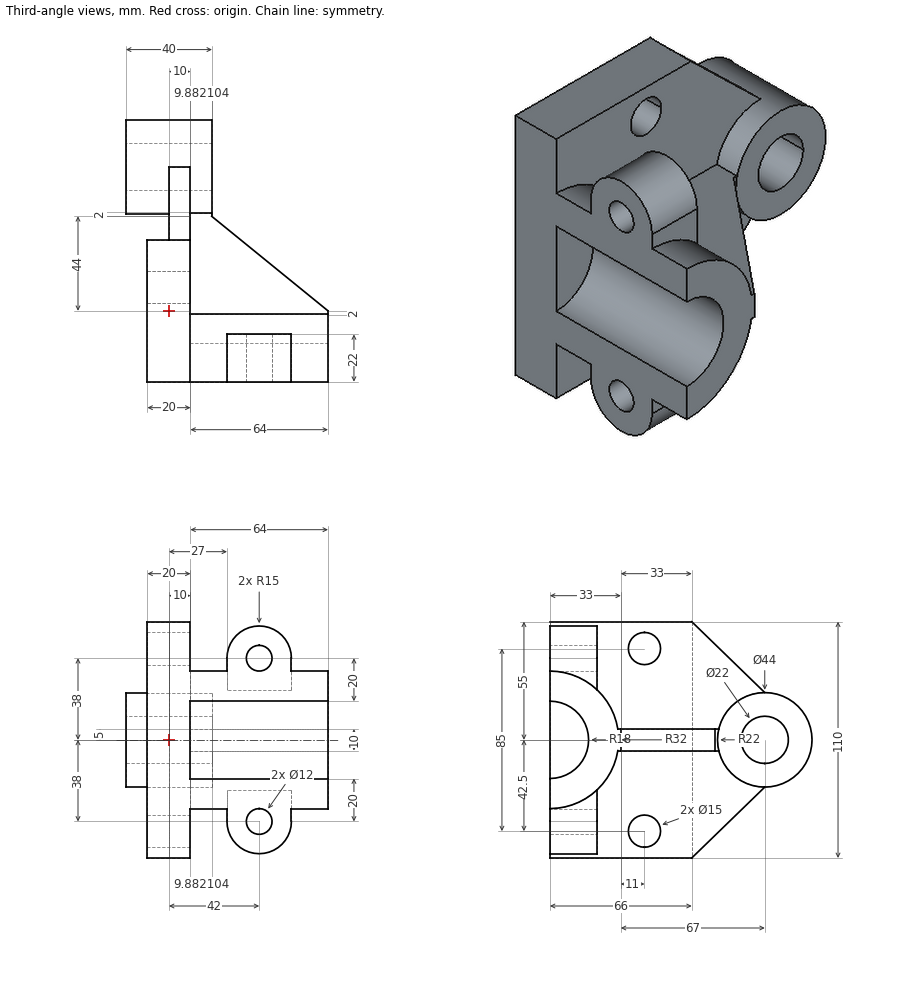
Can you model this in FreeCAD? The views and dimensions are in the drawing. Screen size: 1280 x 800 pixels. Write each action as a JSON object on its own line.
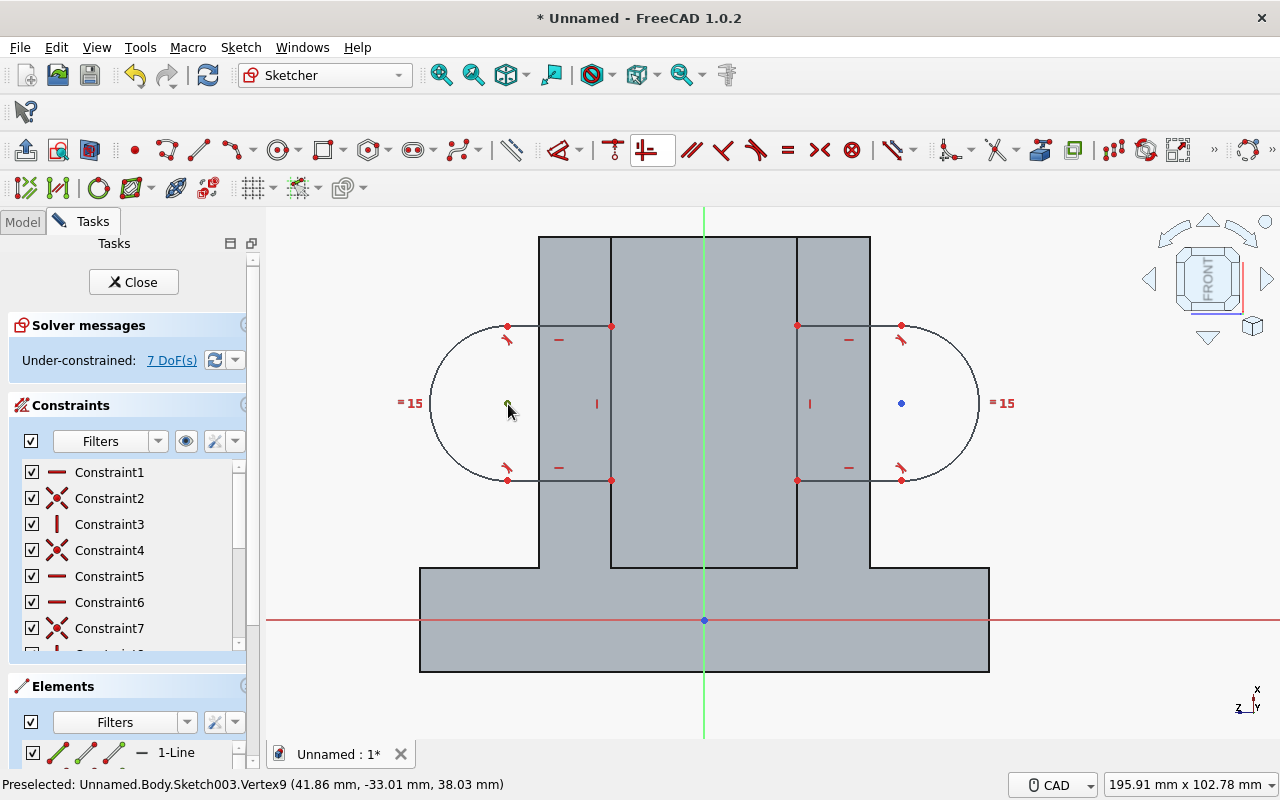
{"action": "left_click", "coordinate": [901, 403]}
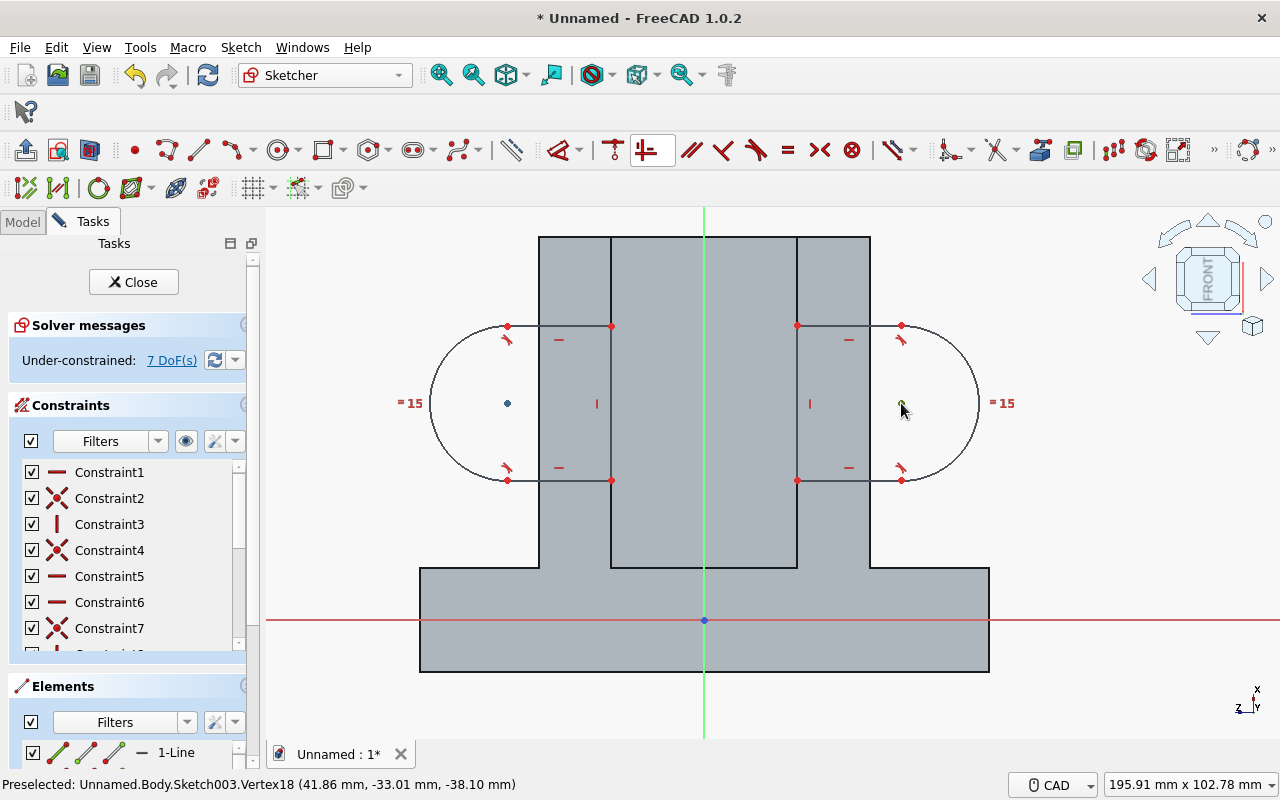
{"action": "left_click", "coordinate": [704, 677]}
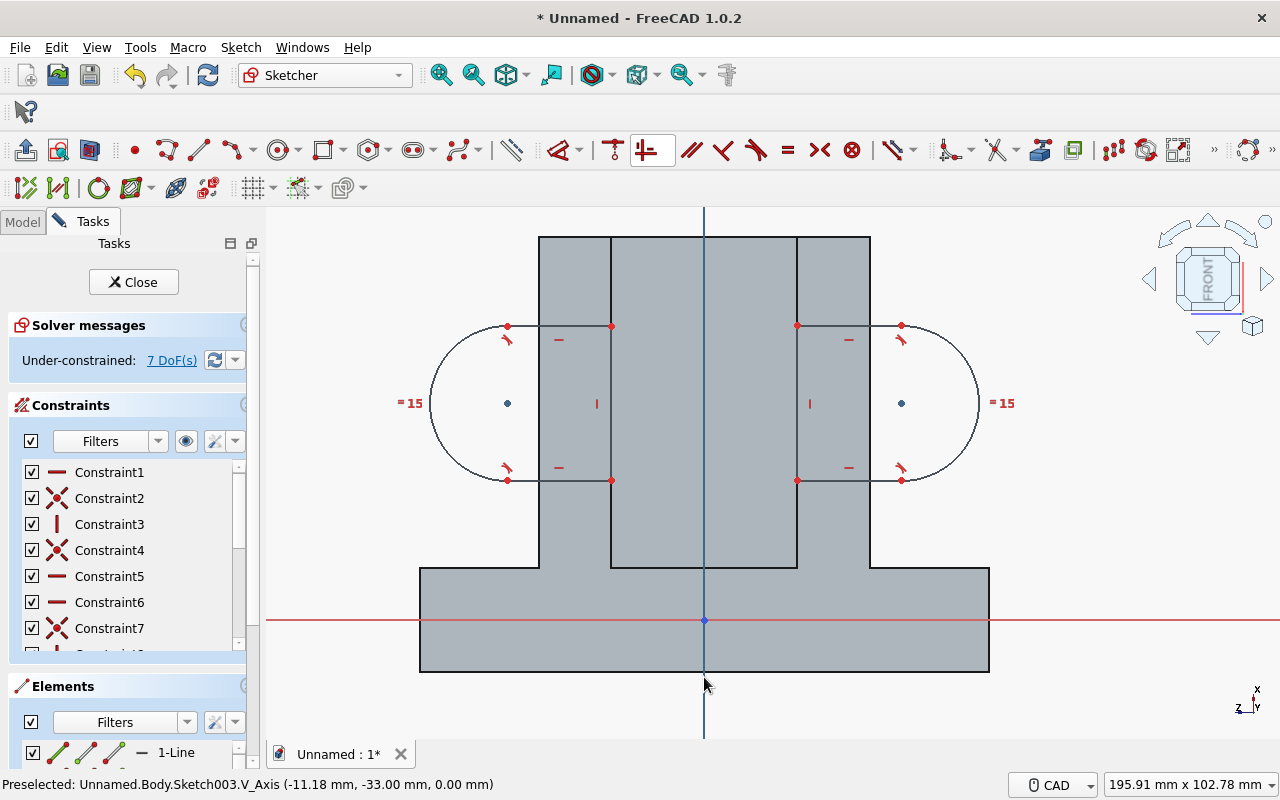
{"action": "left_click", "coordinate": [820, 150]}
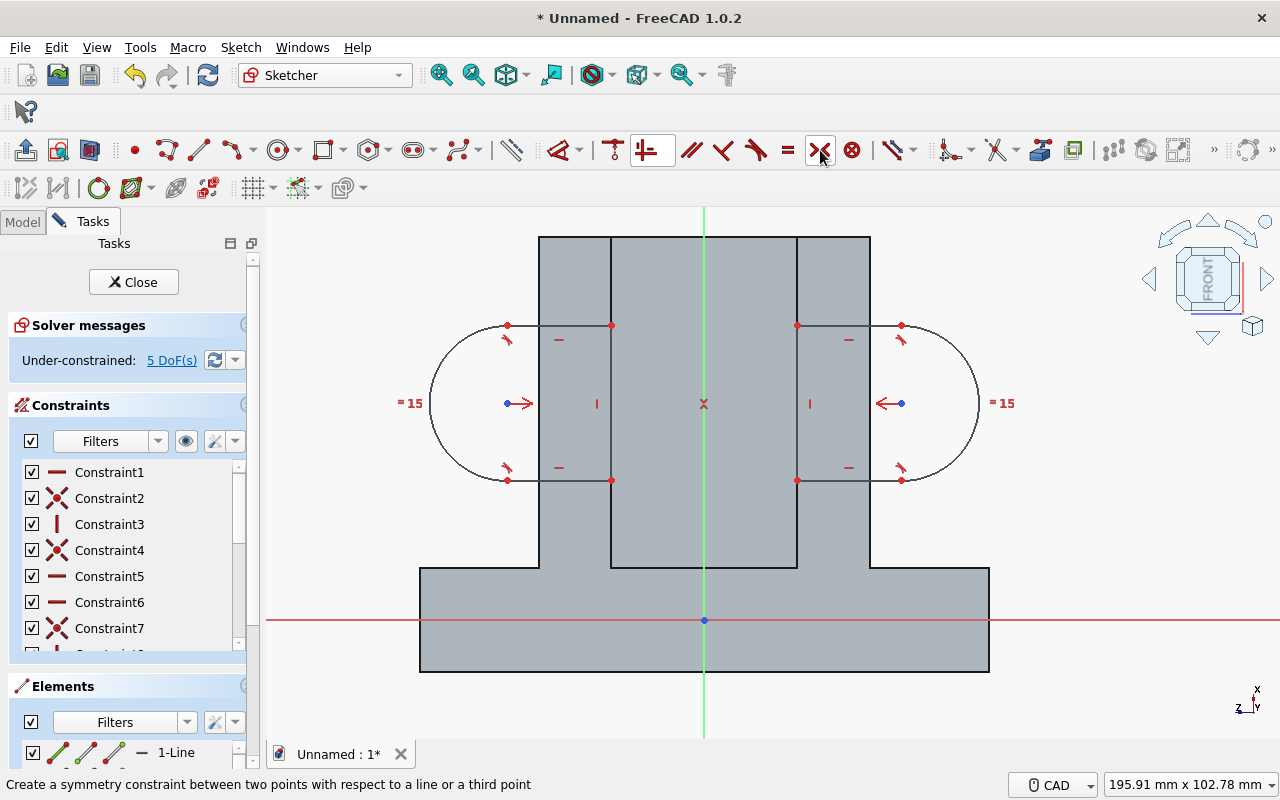
{"action": "left_click", "coordinate": [558, 150]}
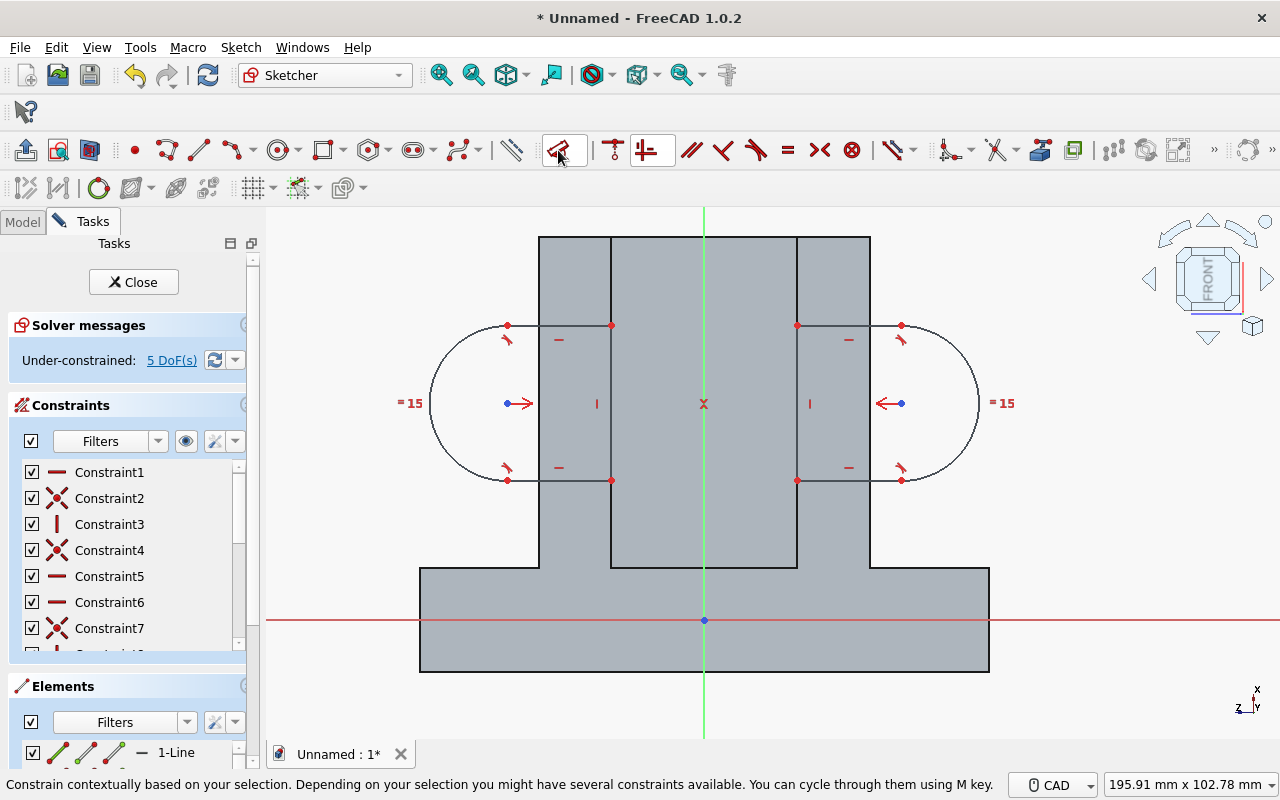
{"action": "left_click", "coordinate": [444, 358]}
{"action": "left_click", "coordinate": [418, 339]}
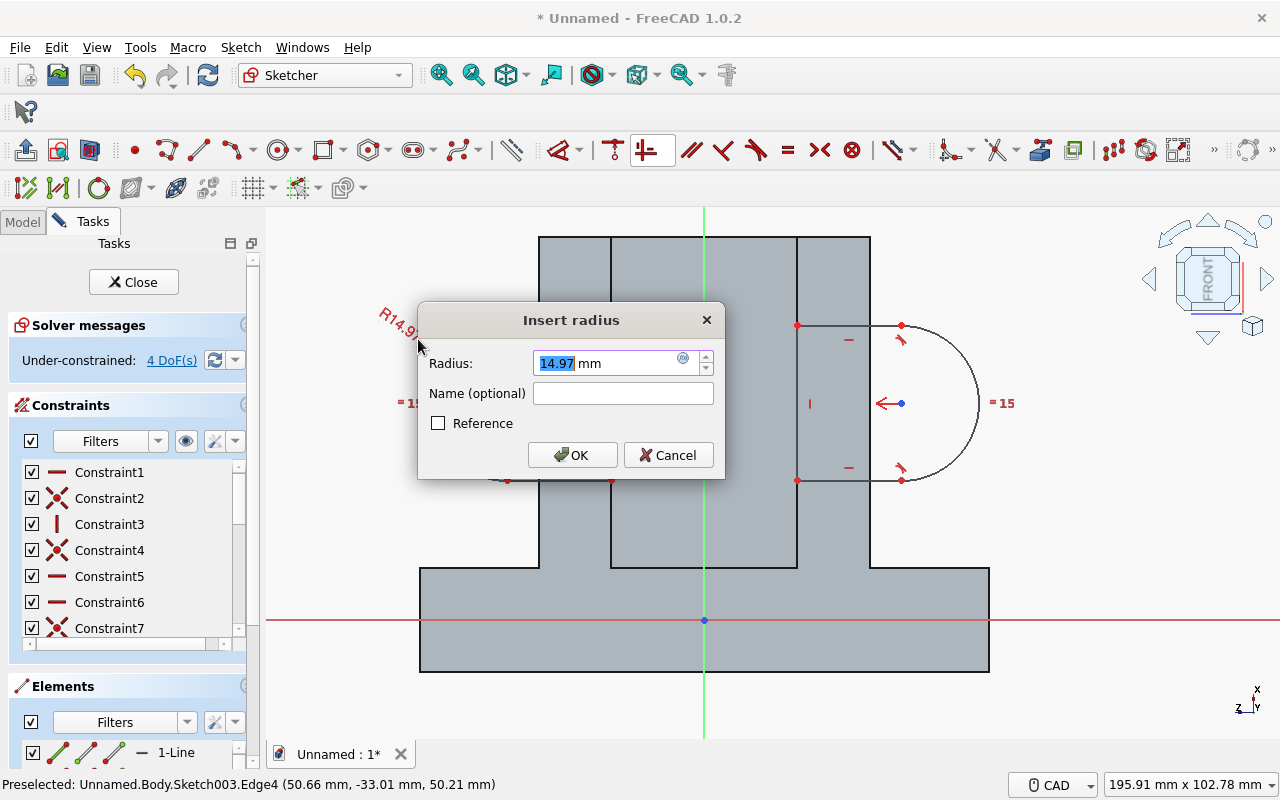
{"action": "type", "text": "15"}
{"action": "key", "text": "Return"}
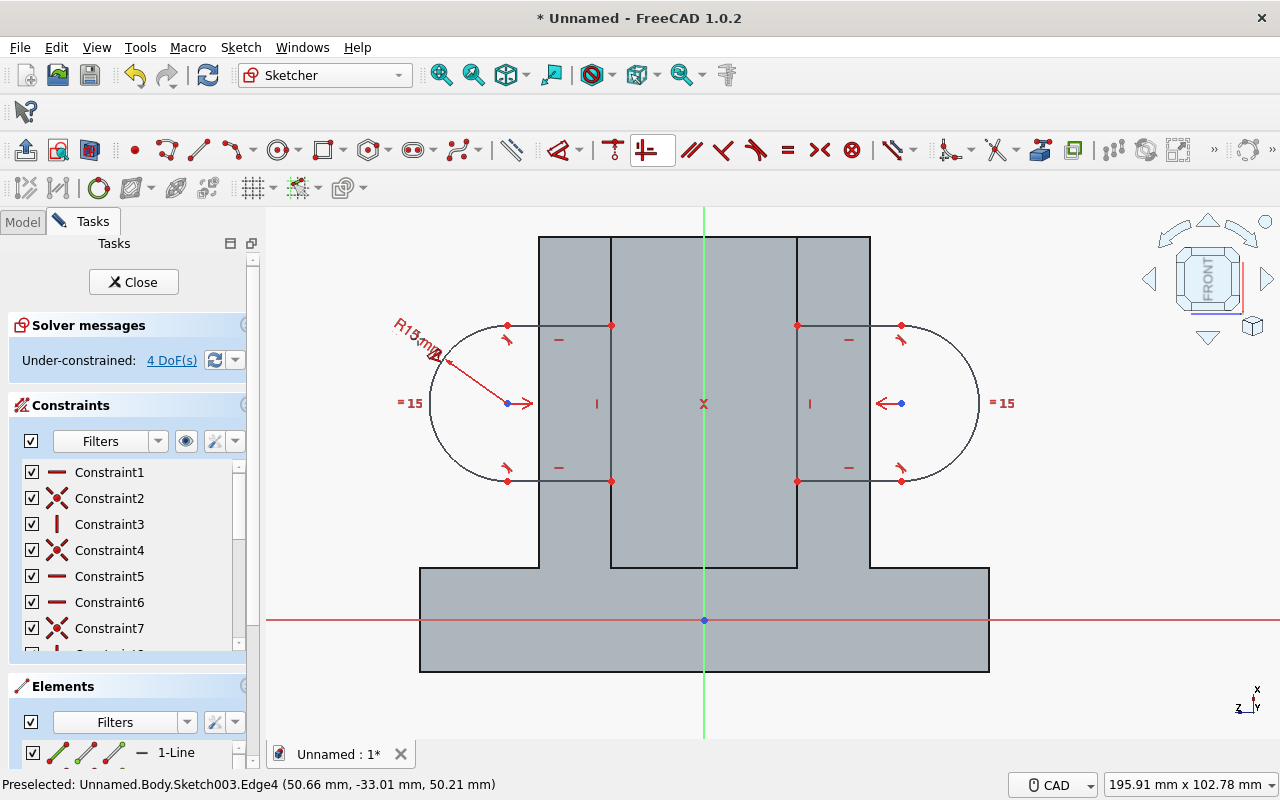
{"action": "left_click", "coordinate": [538, 481]}
{"action": "left_click", "coordinate": [559, 515]}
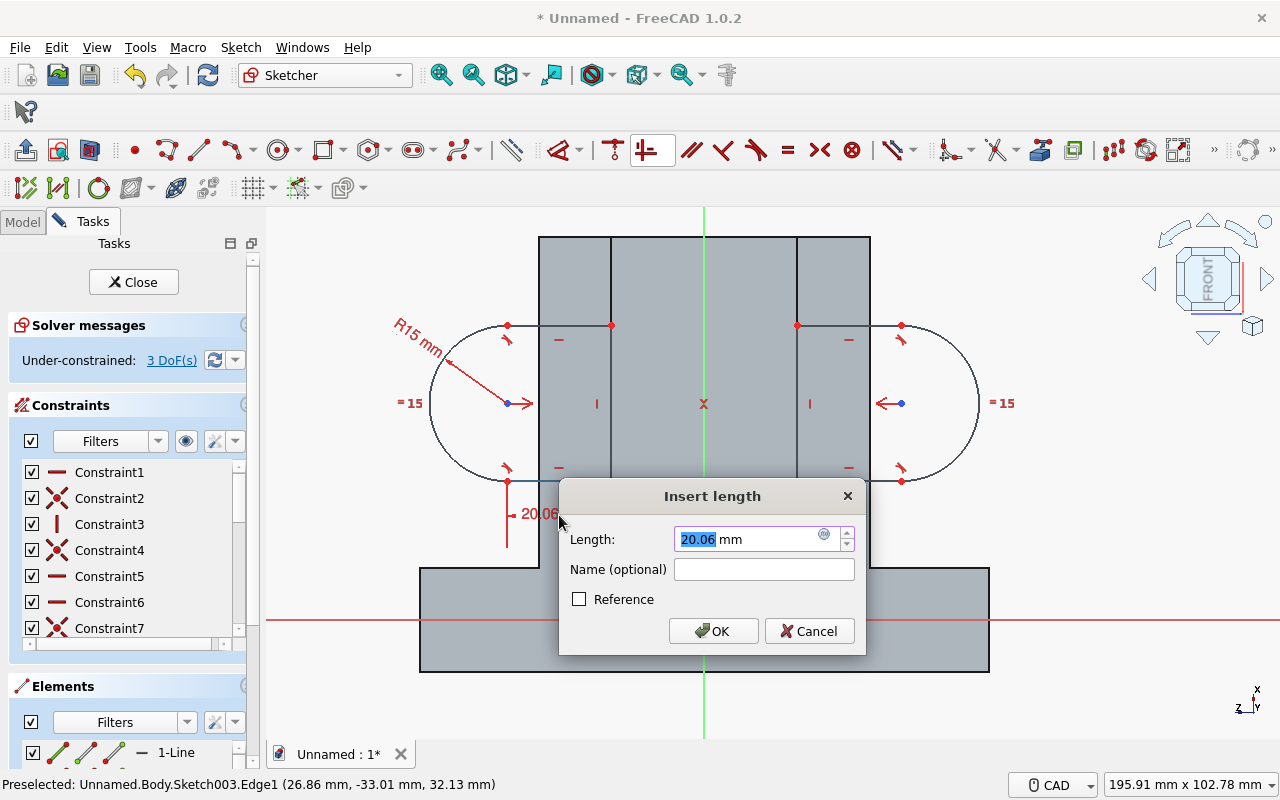
{"action": "type", "text": "20"}
{"action": "key", "text": "Return"}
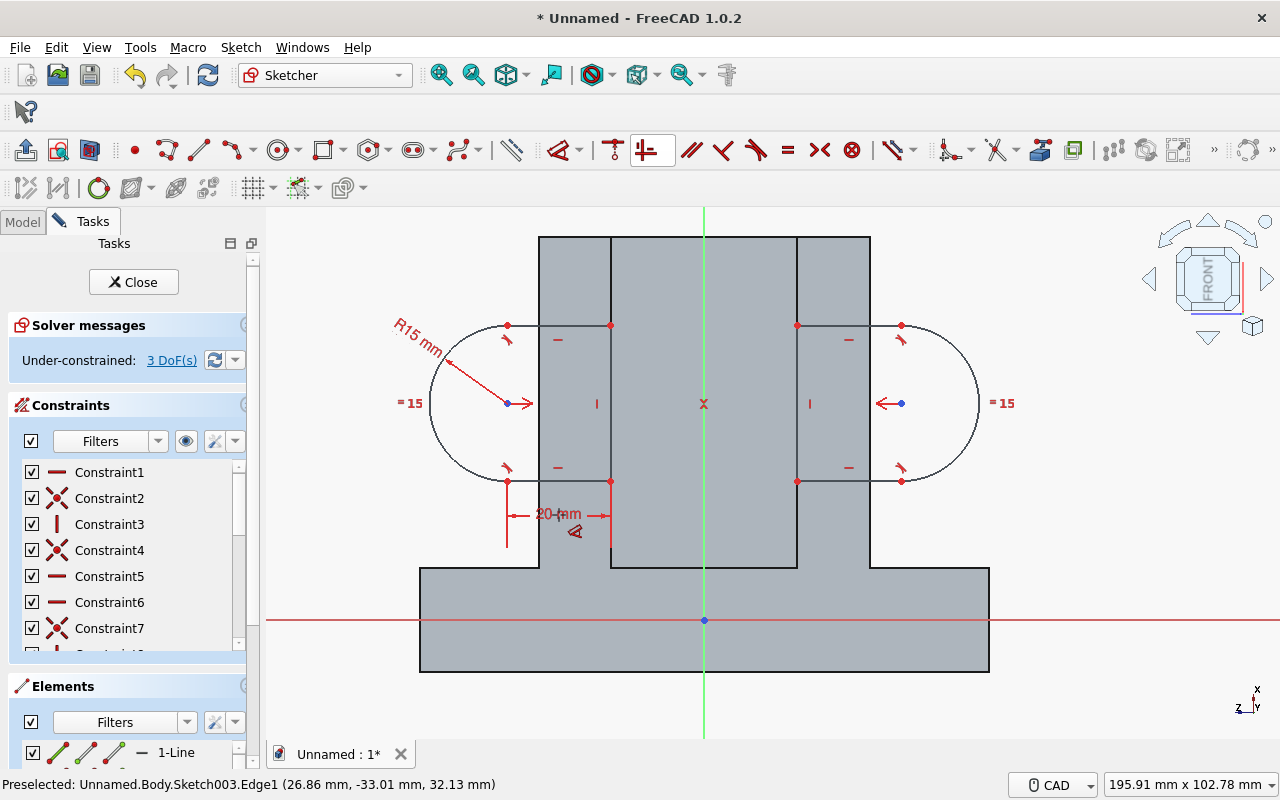
{"action": "left_click", "coordinate": [870, 326]}
{"action": "left_click", "coordinate": [849, 292]}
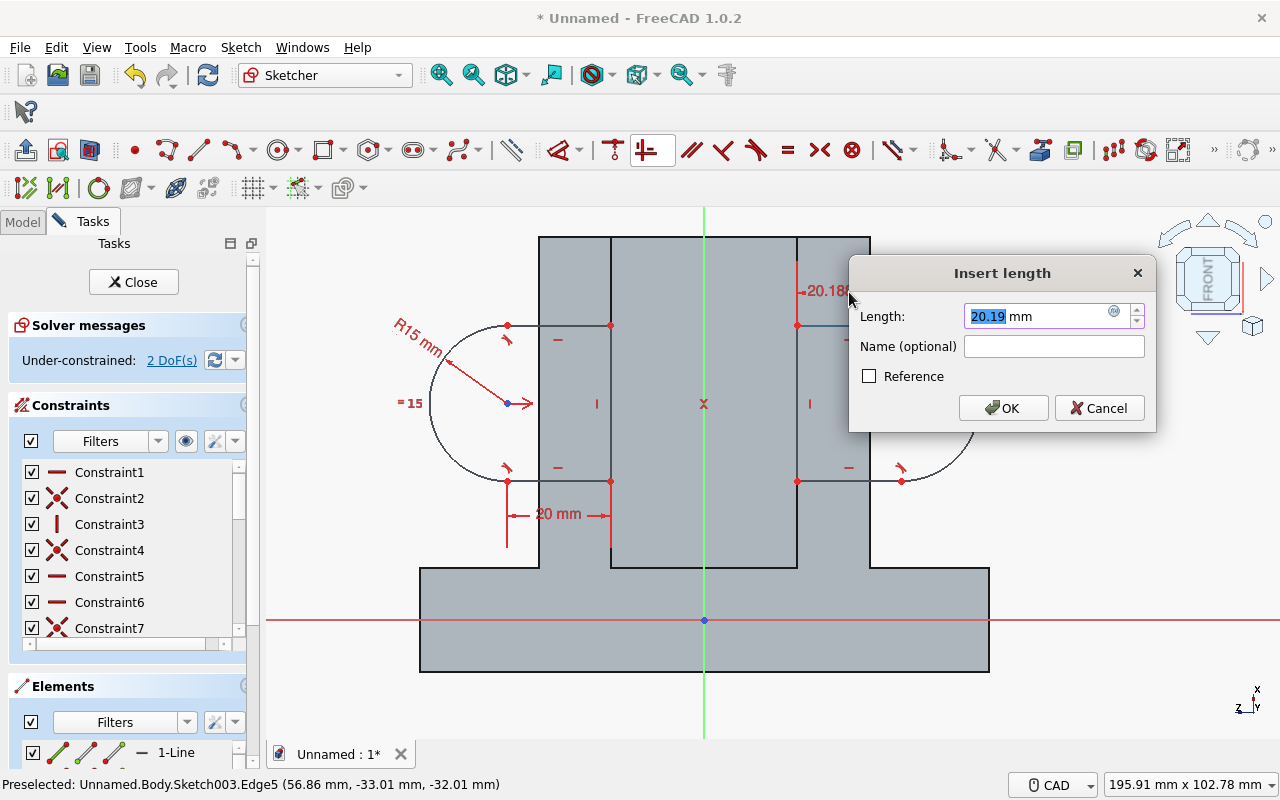
{"action": "type", "text": "20"}
{"action": "key", "text": "Return"}